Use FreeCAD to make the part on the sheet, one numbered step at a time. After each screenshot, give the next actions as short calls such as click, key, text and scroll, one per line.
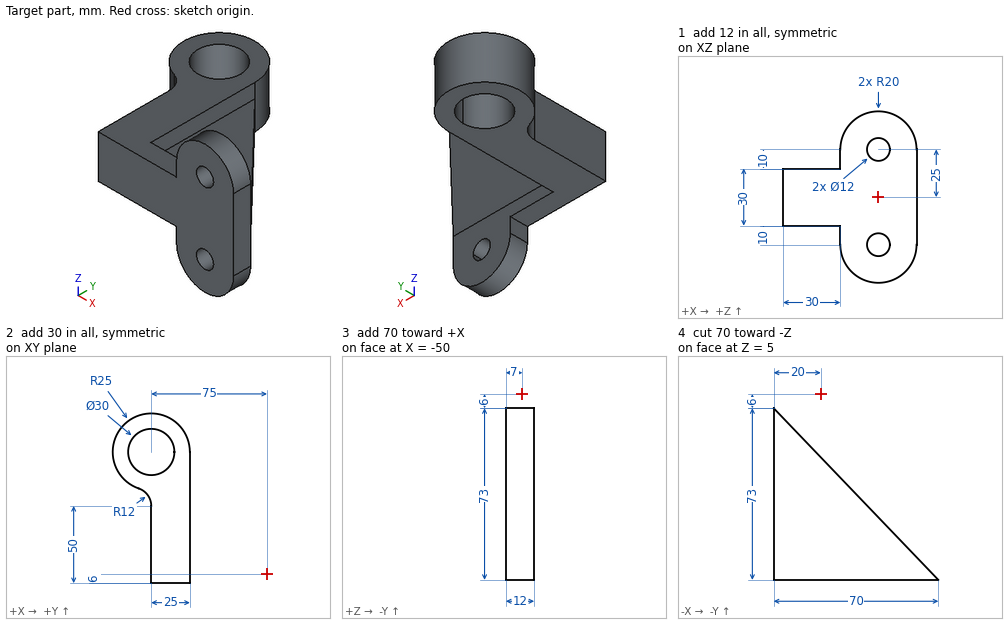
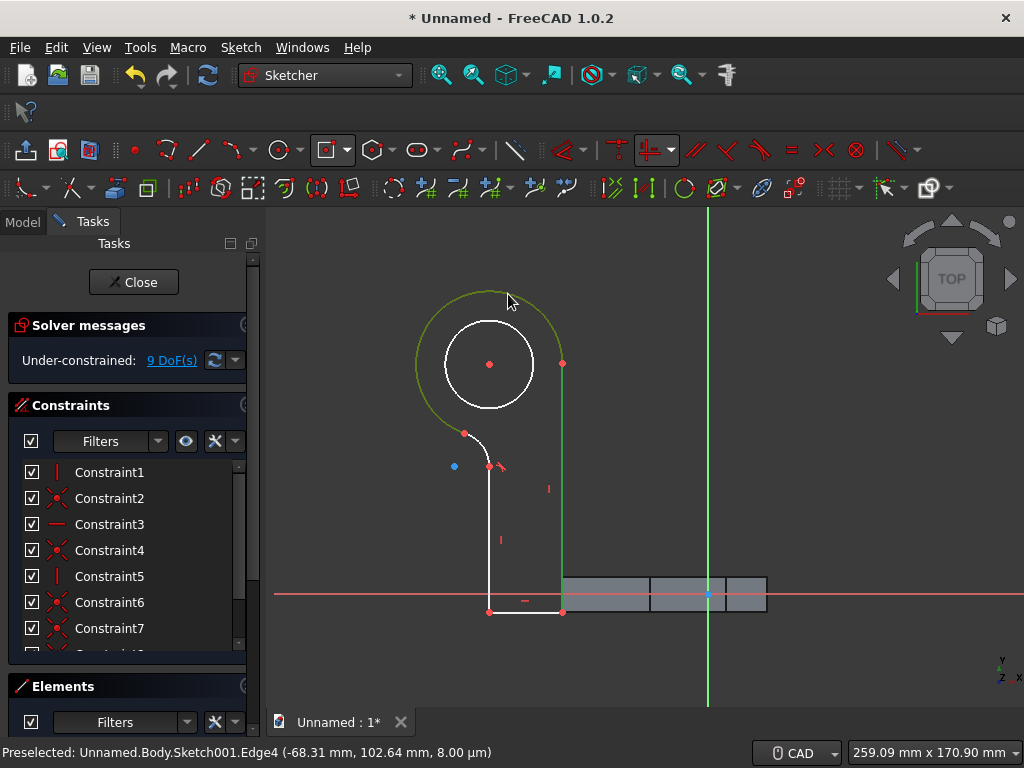
click(760, 150)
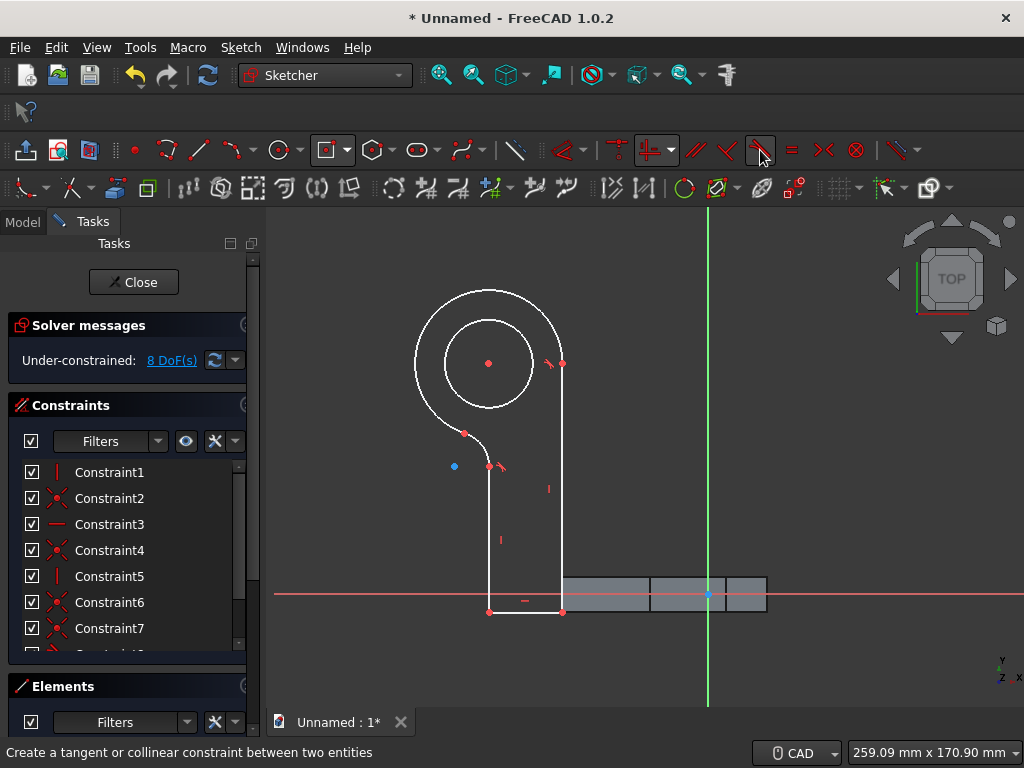
click(508, 293)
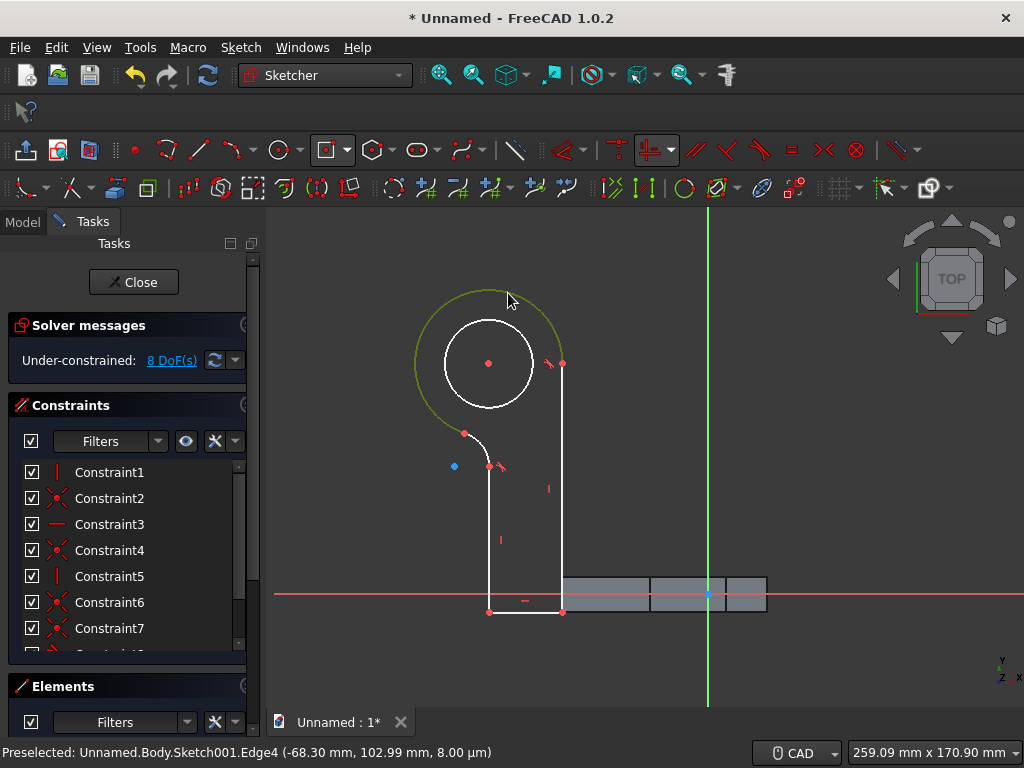
click(487, 454)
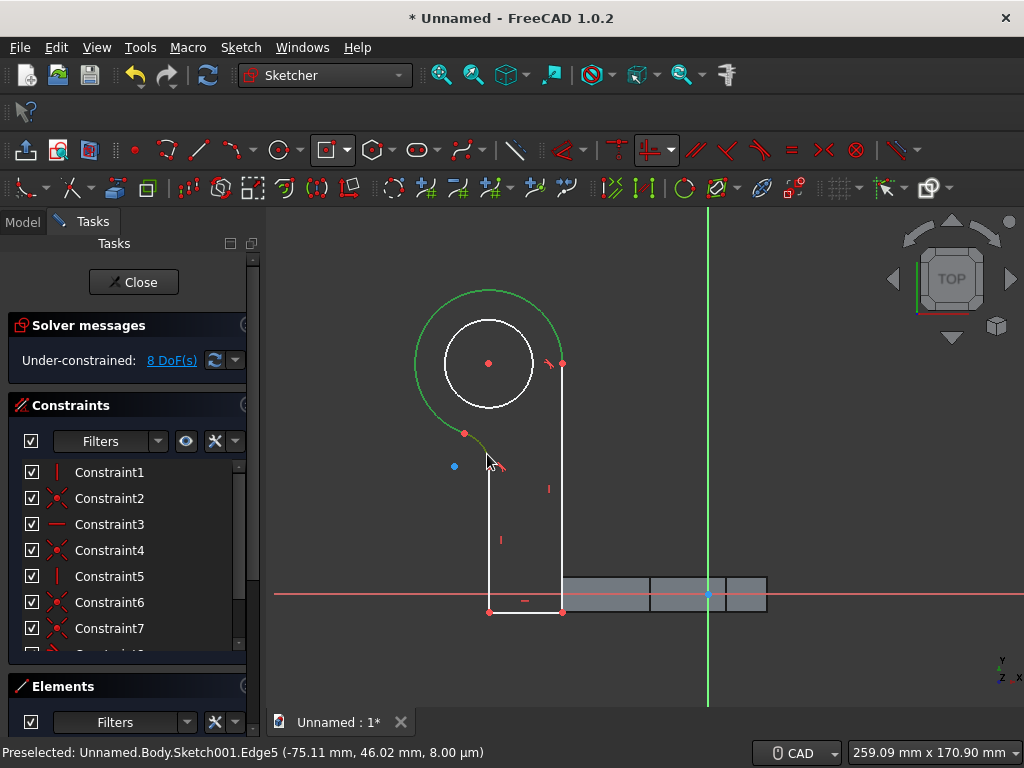
click(760, 150)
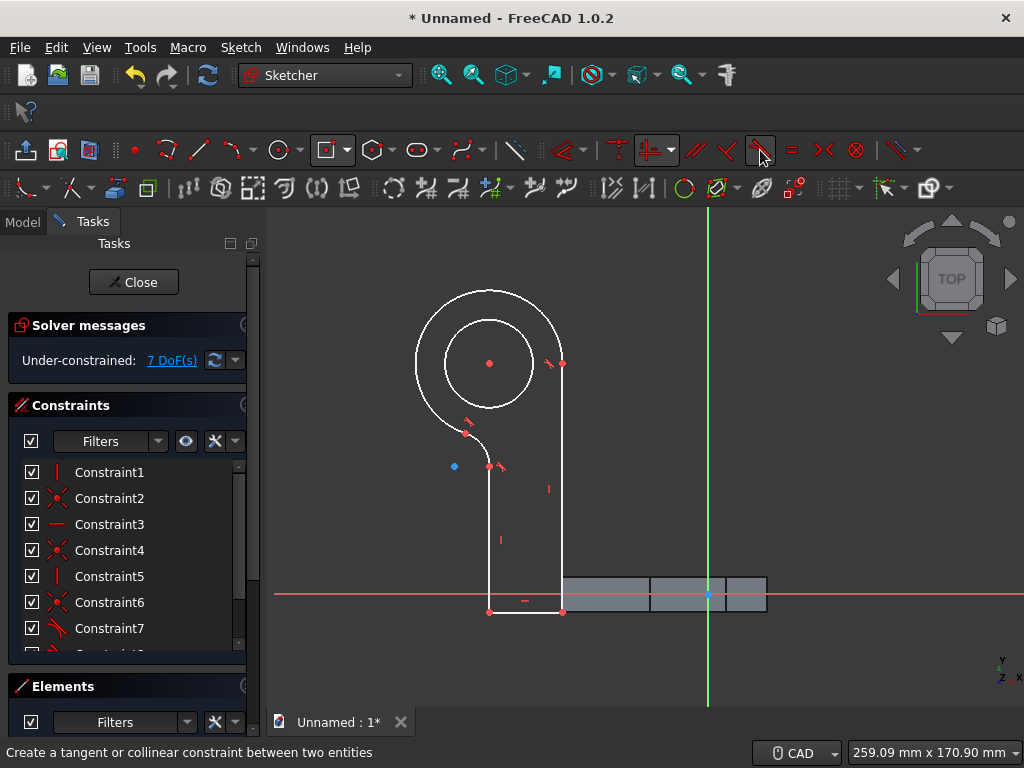
click(562, 150)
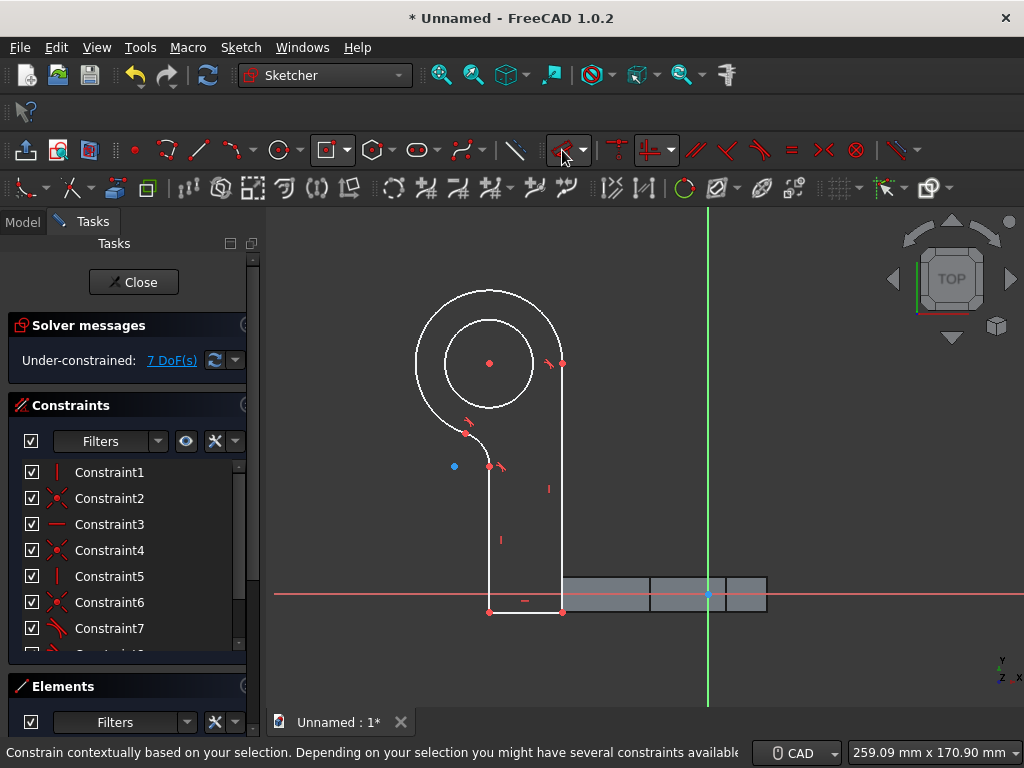
click(507, 293)
click(515, 262)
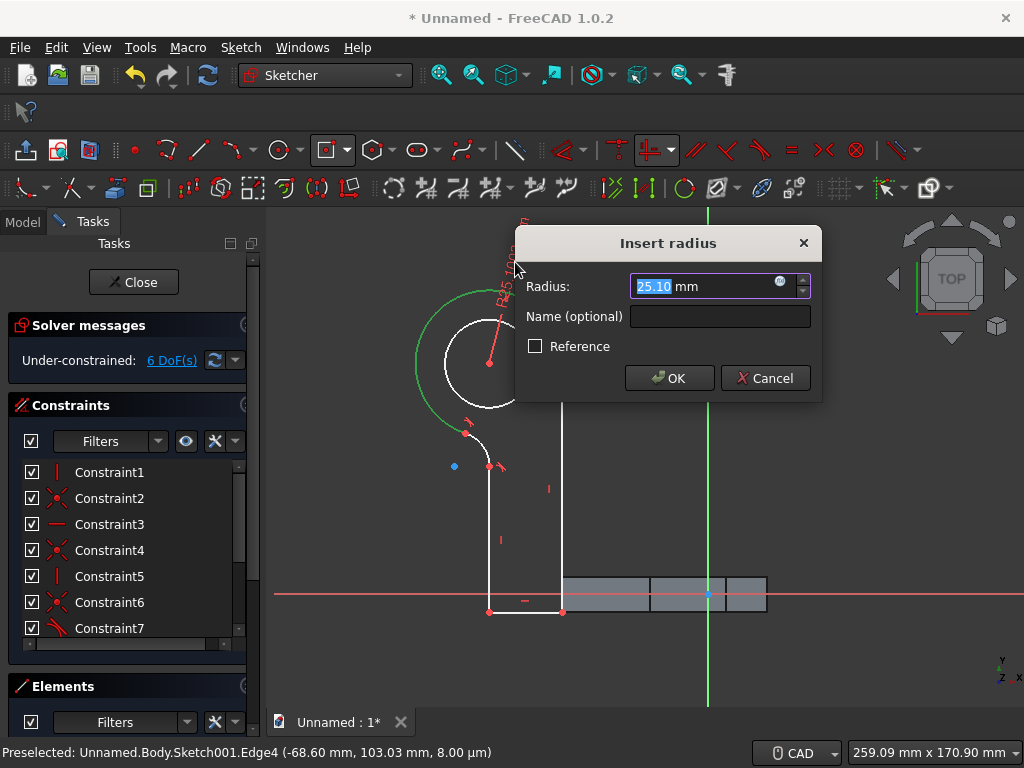
text(25)
key(Return)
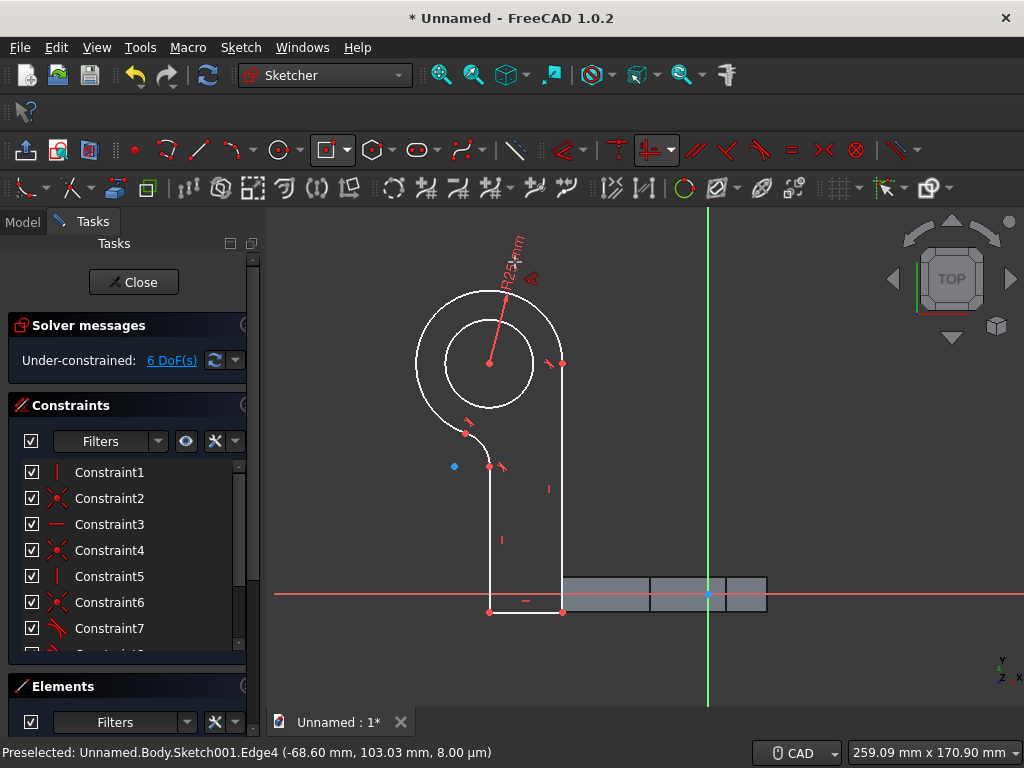
click(487, 454)
click(517, 443)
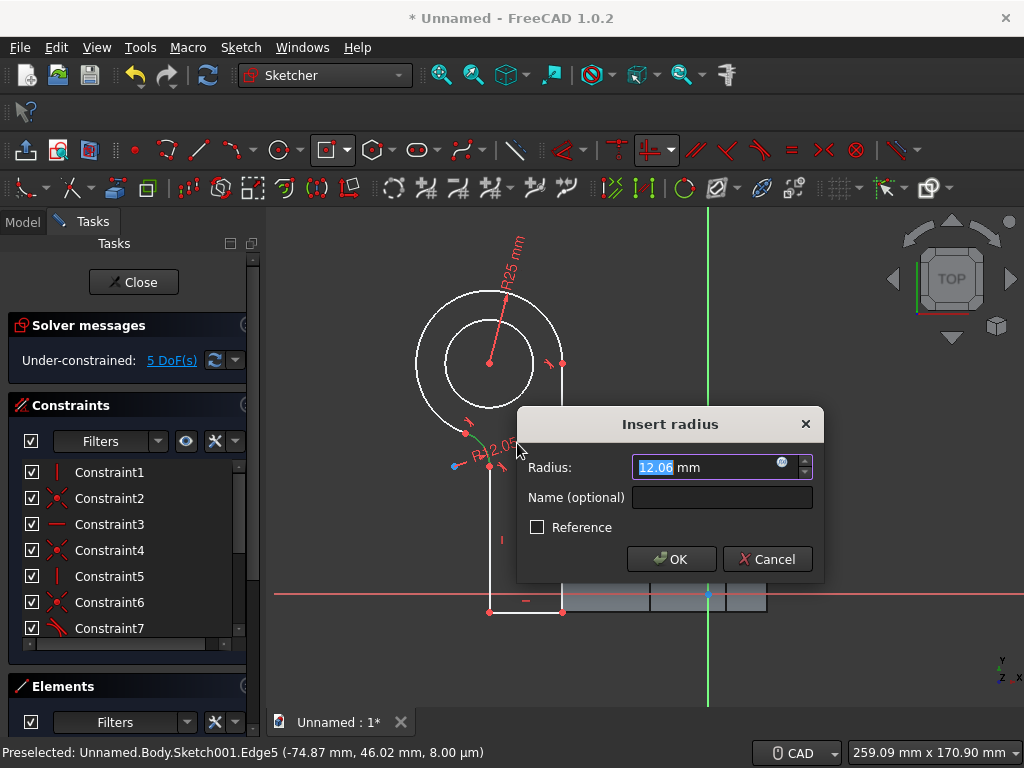
text(12)
key(Return)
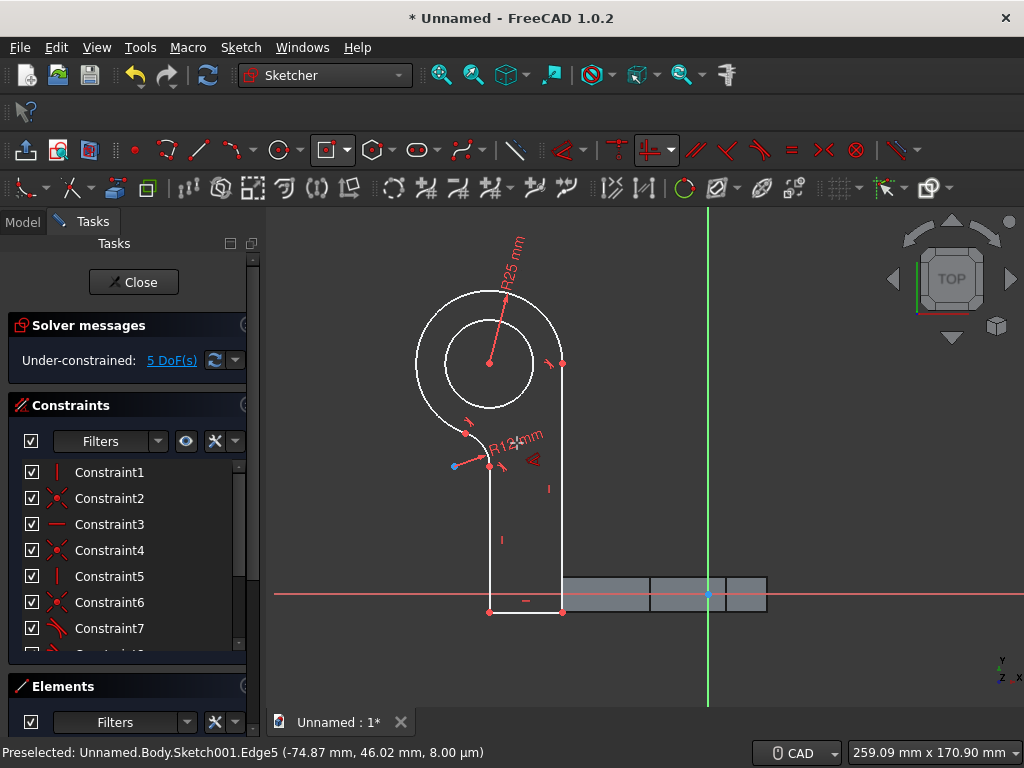
click(520, 333)
click(543, 417)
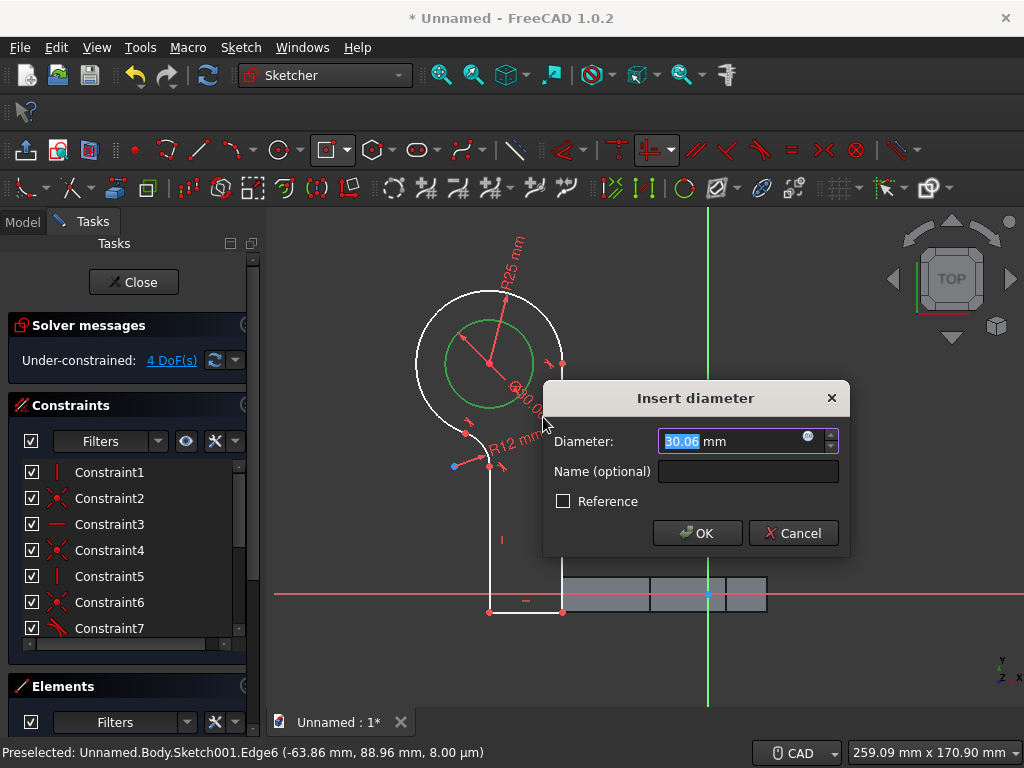
text(30)
key(Return)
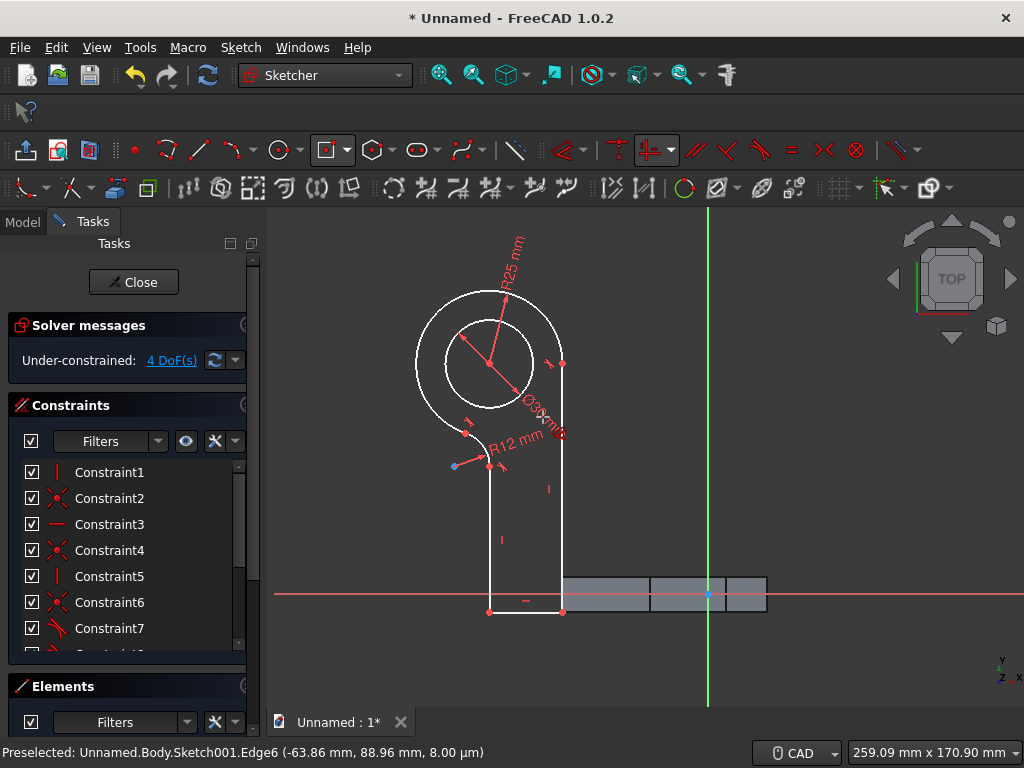
click(490, 510)
click(456, 540)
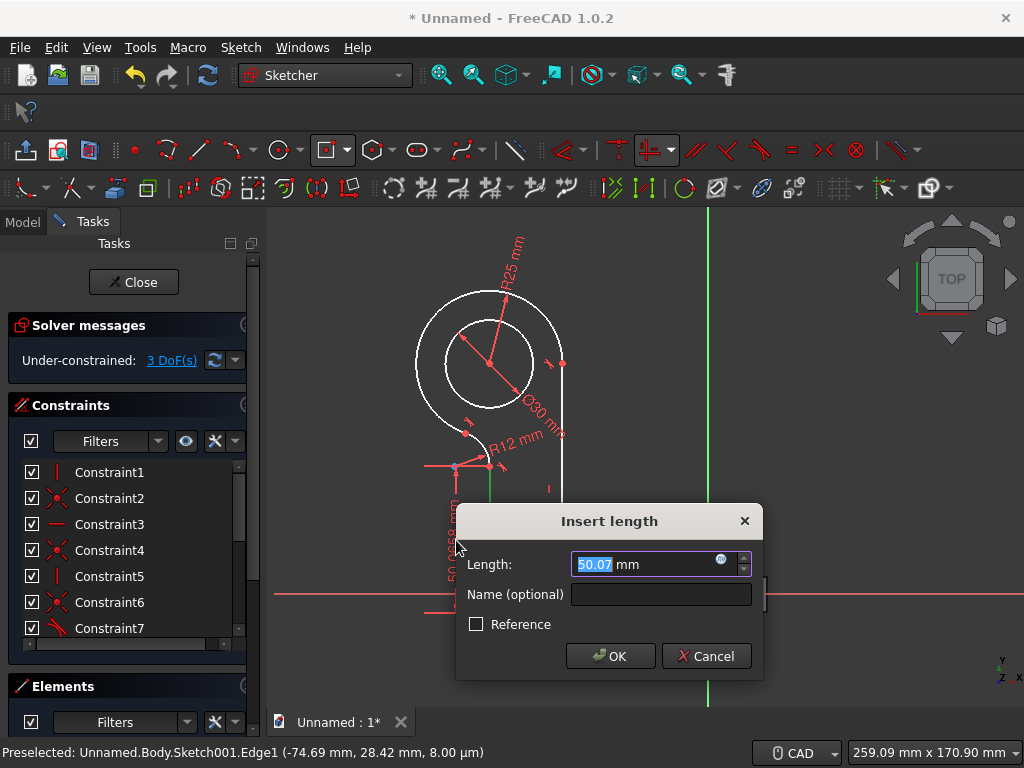
text(50)
key(Return)